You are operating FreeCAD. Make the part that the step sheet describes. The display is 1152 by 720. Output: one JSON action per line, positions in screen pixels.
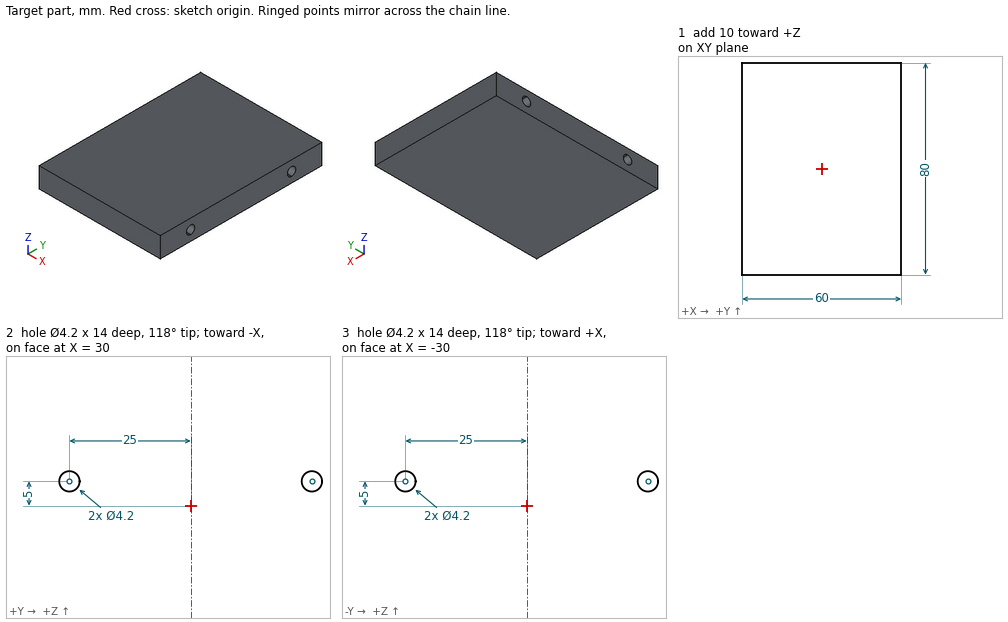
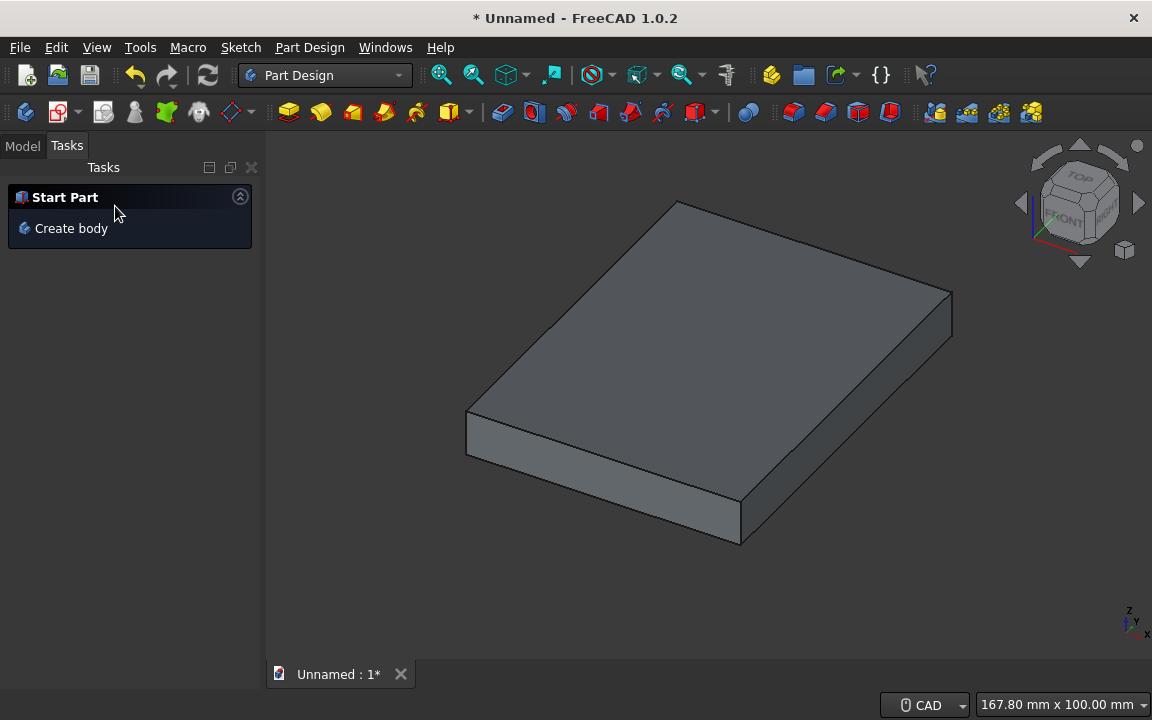
{"action": "left_click", "coordinate": [937, 328]}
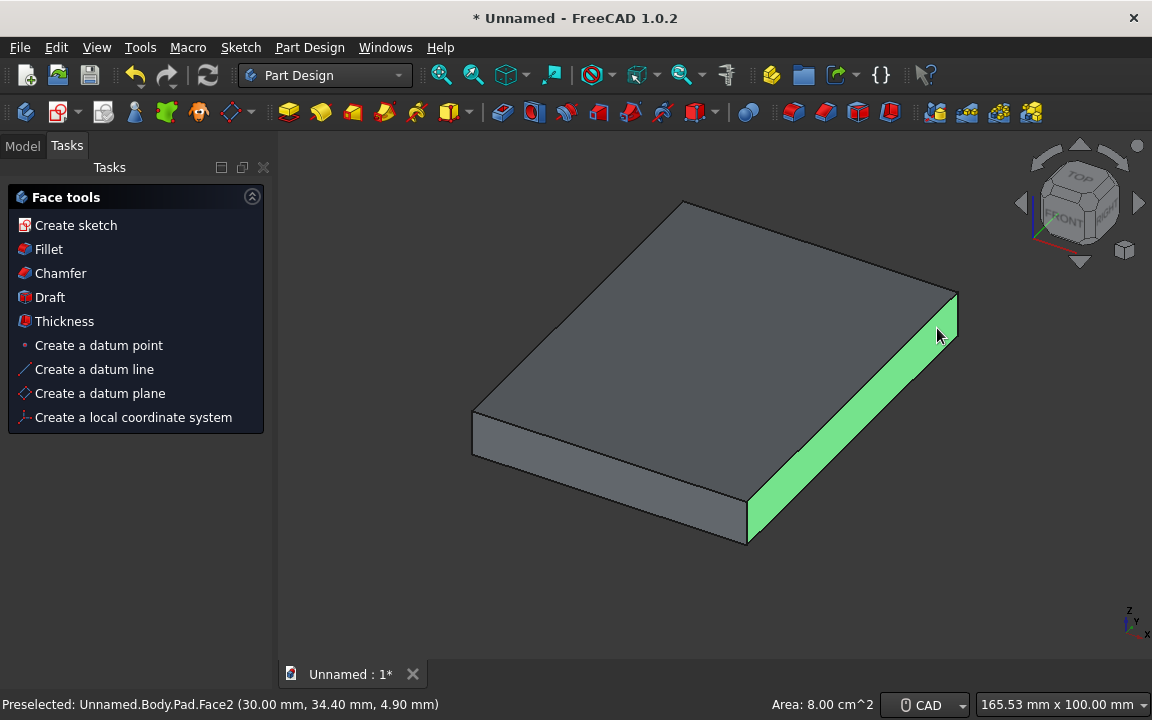
{"action": "left_click", "coordinate": [58, 112]}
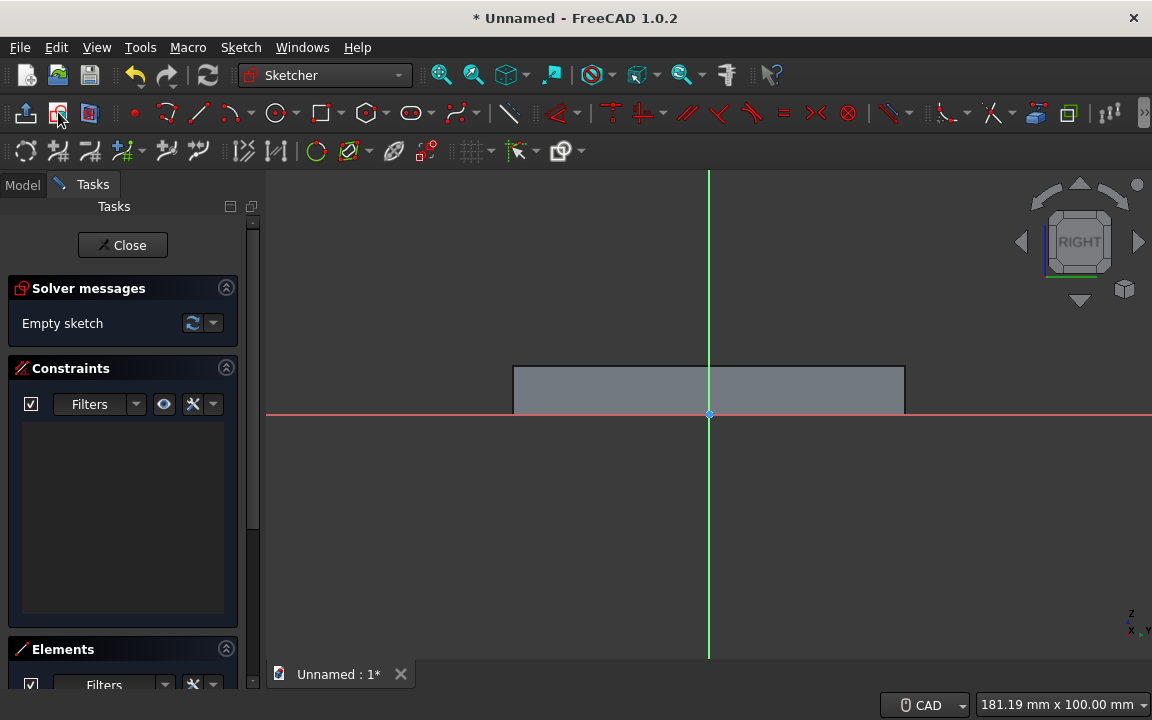
{"action": "scroll", "coordinate": [792, 376], "scroll_direction": "up", "scroll_amount": 3}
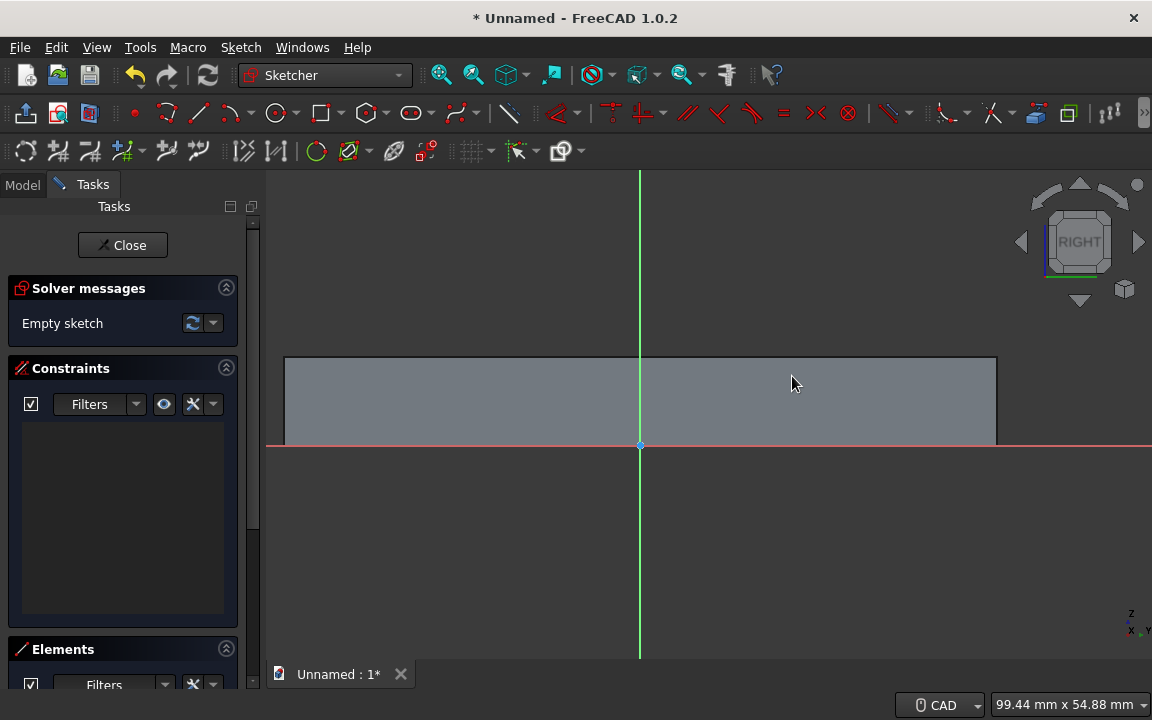
{"action": "left_click", "coordinate": [276, 114]}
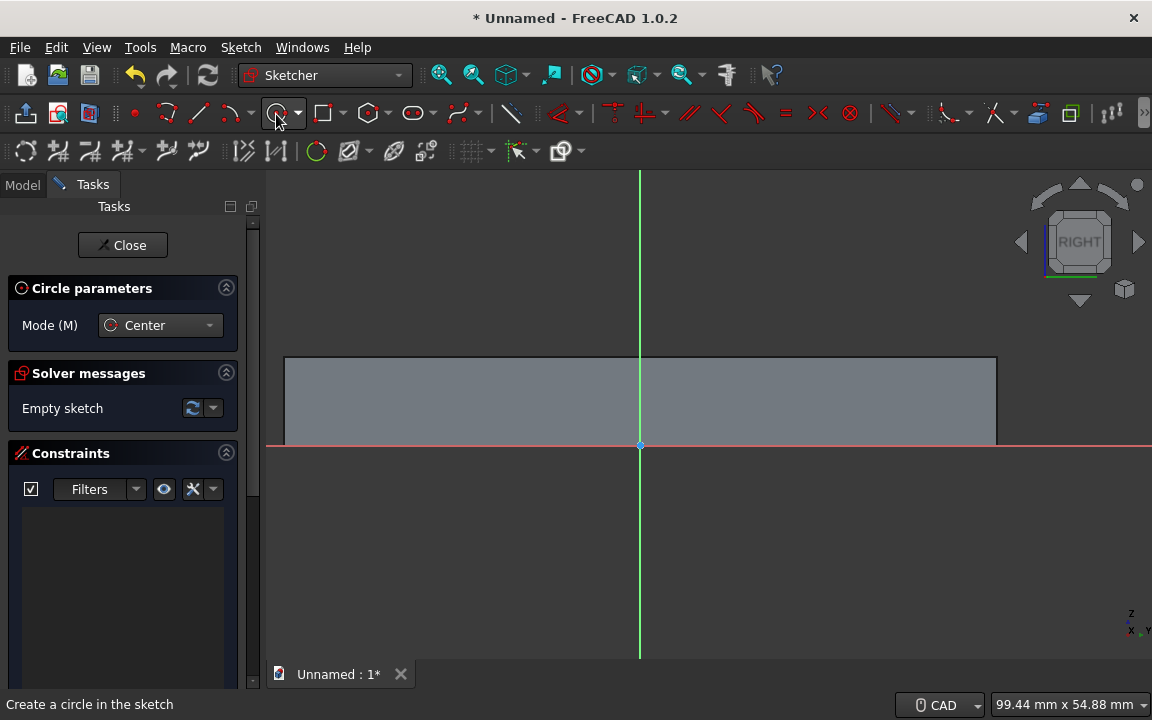
{"action": "left_click", "coordinate": [418, 401]}
{"action": "mouse_move", "coordinate": [431, 388]}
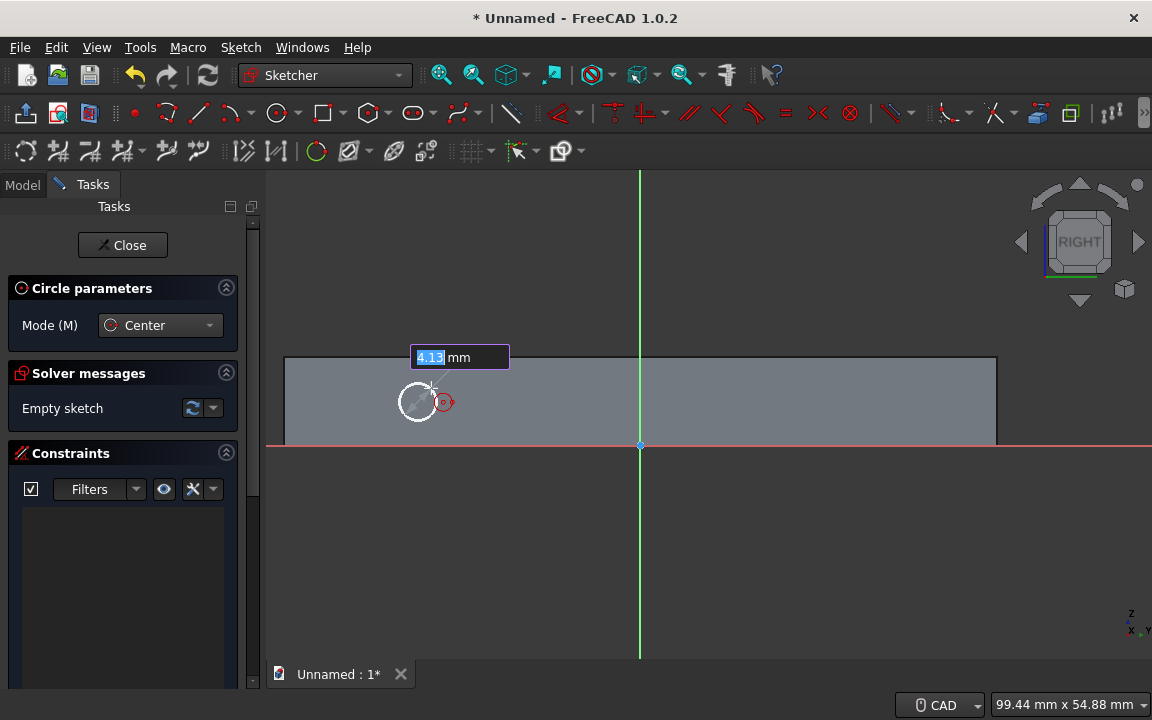
{"action": "type", "text": "4.2"}
{"action": "key", "text": "Return"}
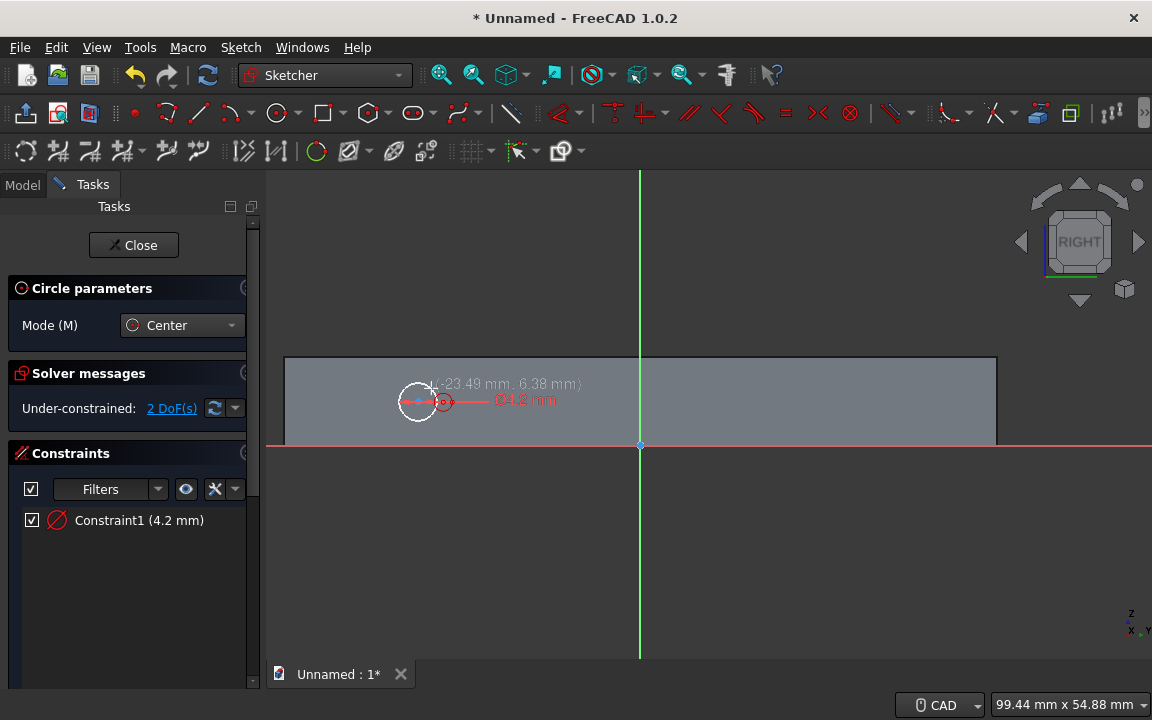
{"action": "left_click", "coordinate": [863, 401]}
{"action": "mouse_move", "coordinate": [876, 388]}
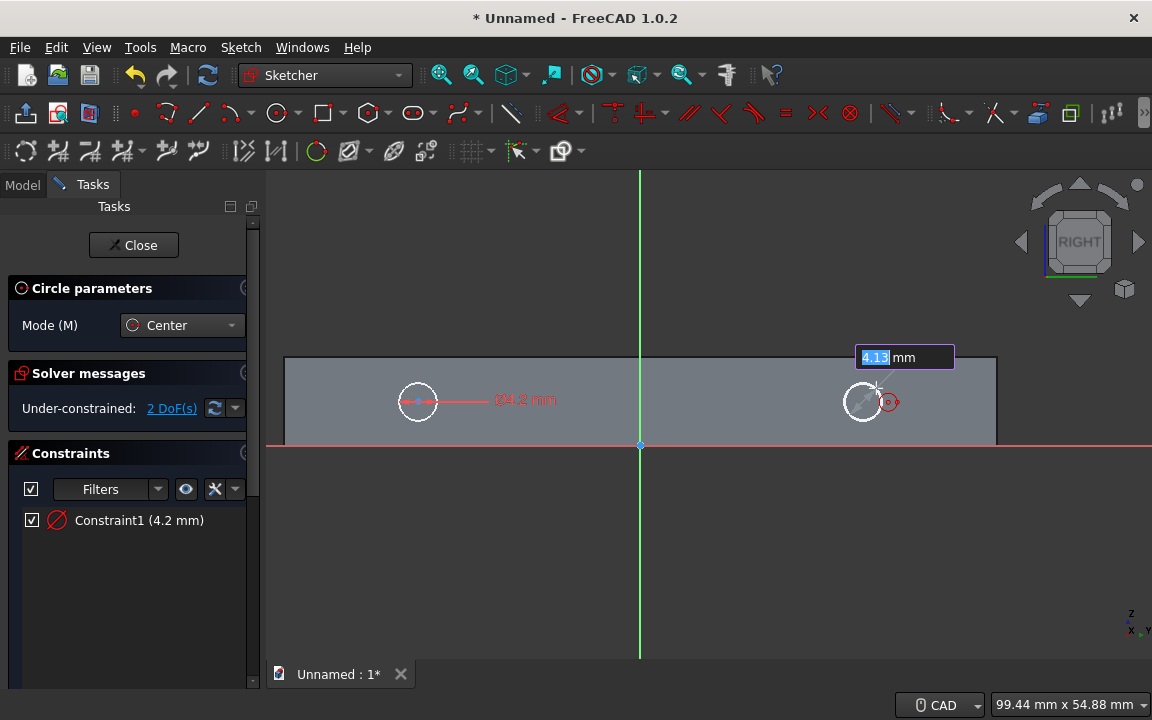
{"action": "type", "text": "4.2"}
{"action": "key", "text": "Return"}
{"action": "key", "text": "Escape"}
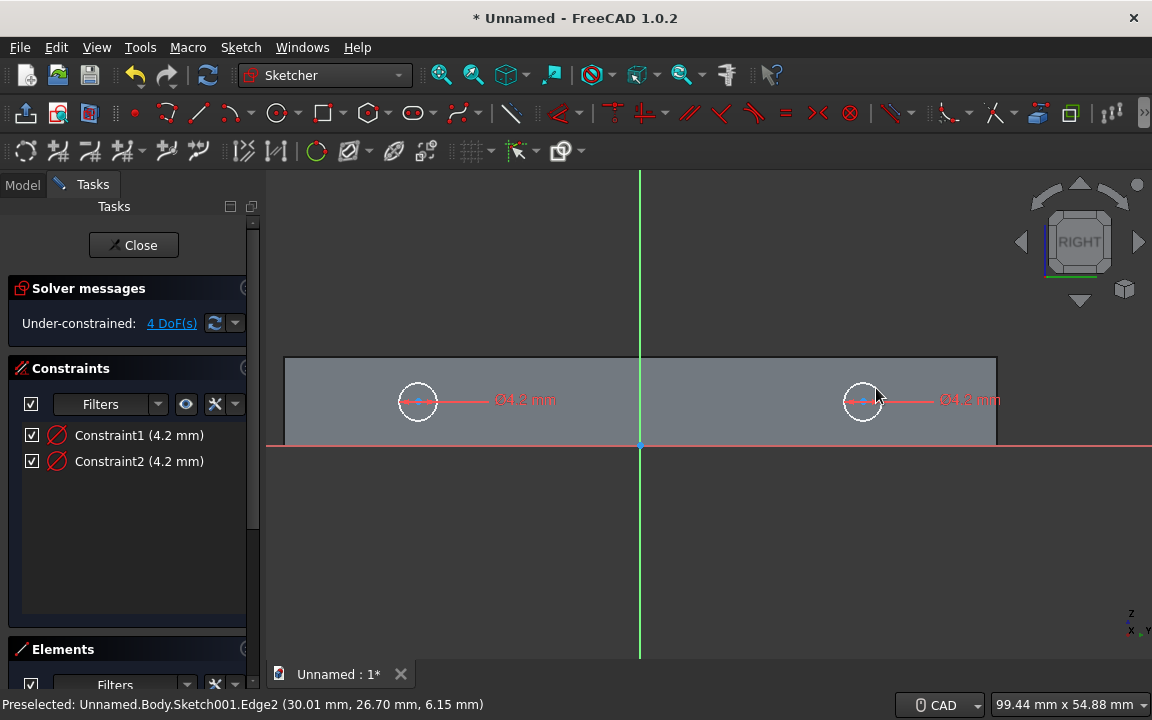
{"action": "left_click", "coordinate": [418, 402]}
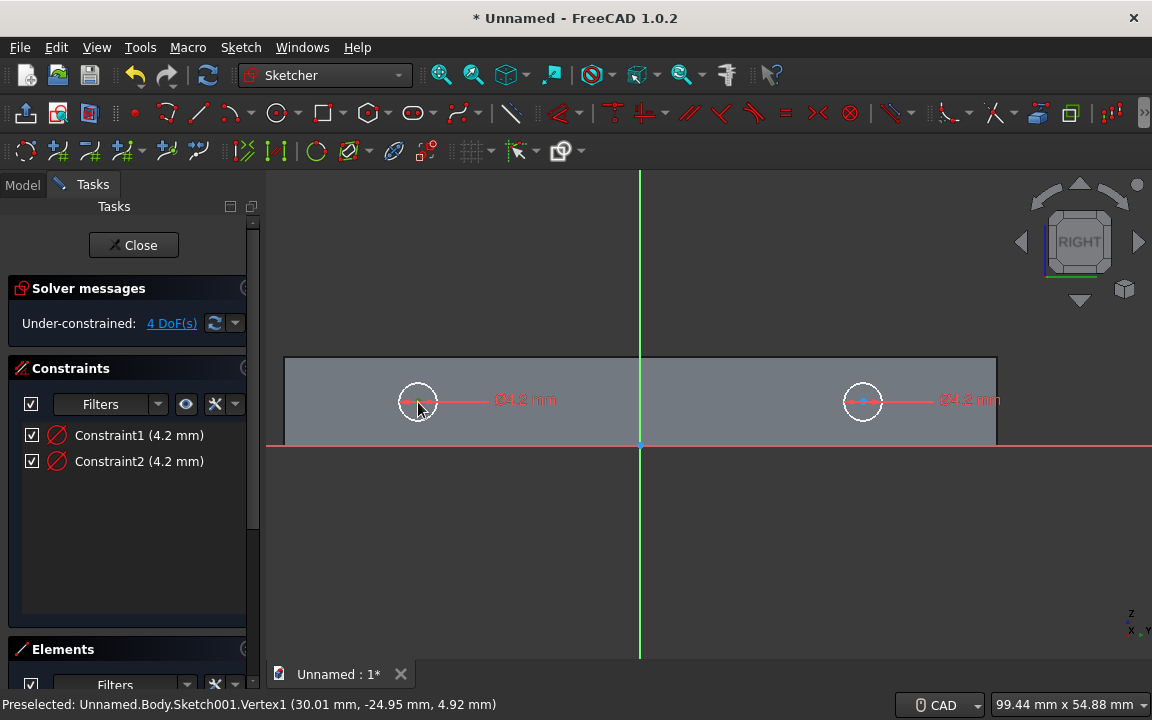
{"action": "left_click", "coordinate": [863, 402]}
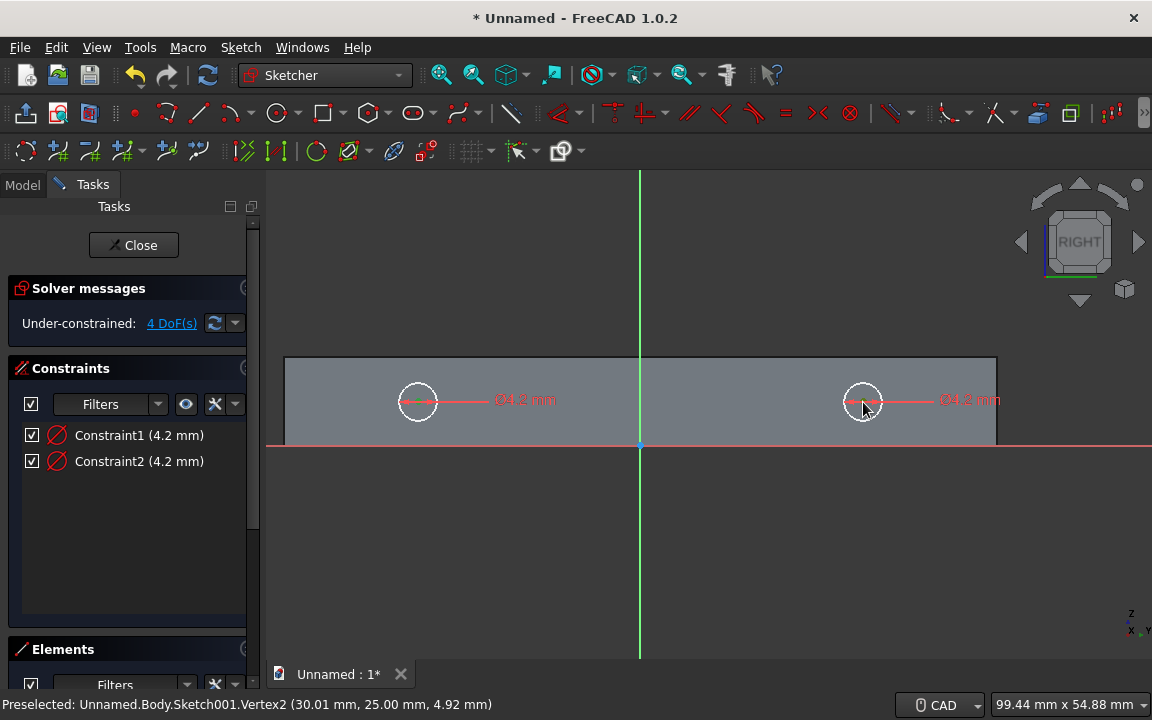
{"action": "left_click", "coordinate": [640, 600]}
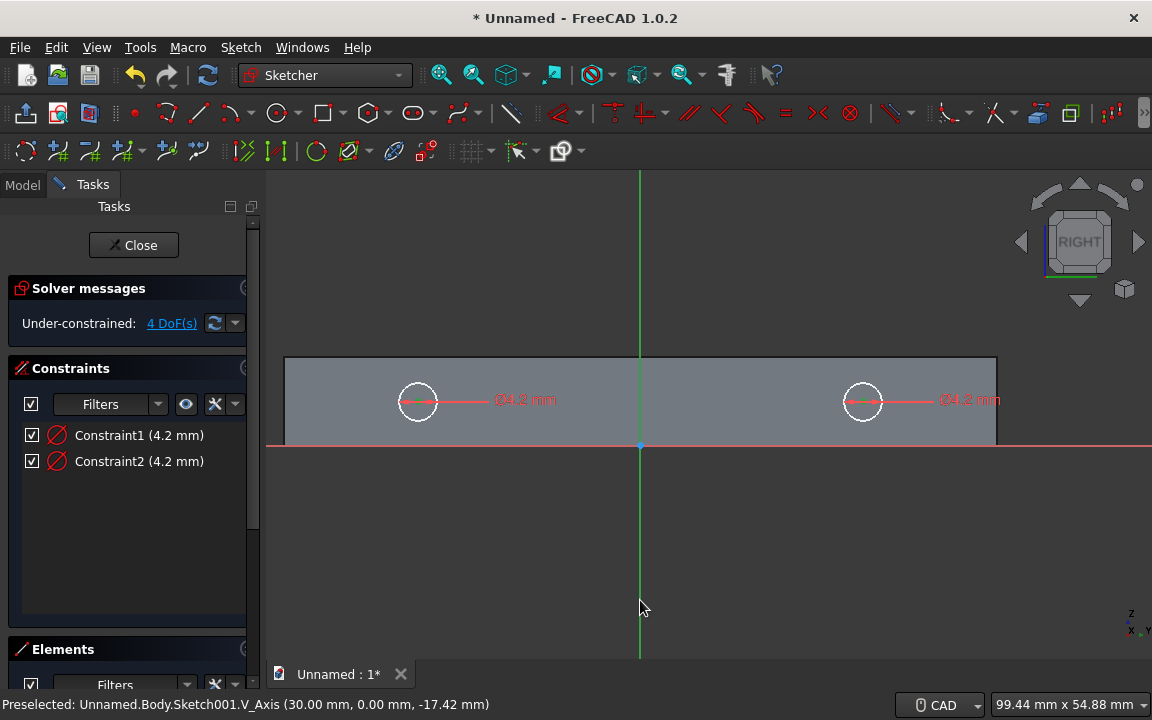
{"action": "left_click", "coordinate": [818, 114]}